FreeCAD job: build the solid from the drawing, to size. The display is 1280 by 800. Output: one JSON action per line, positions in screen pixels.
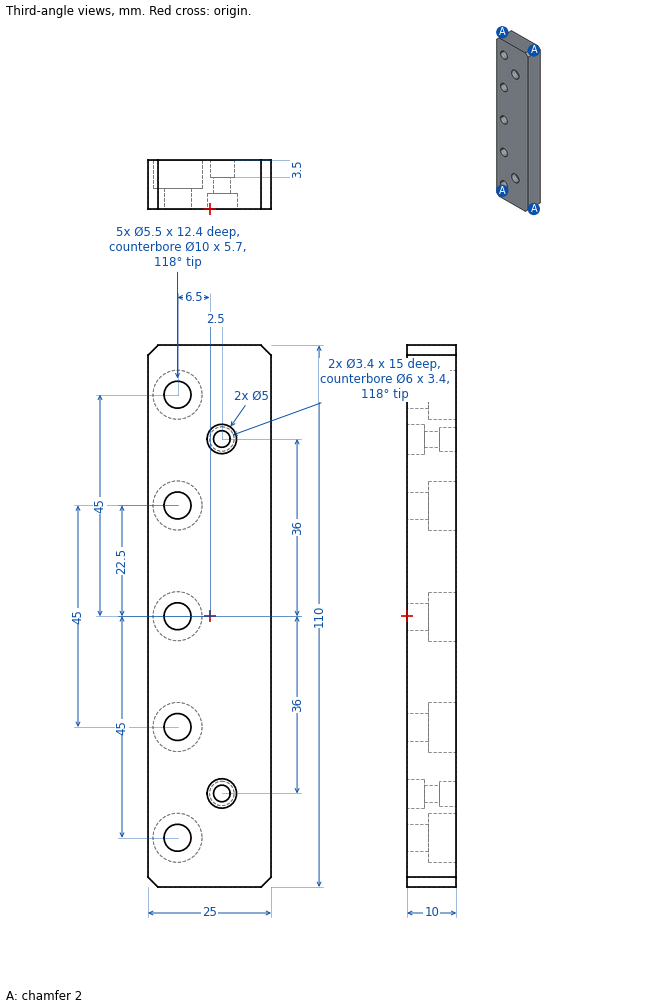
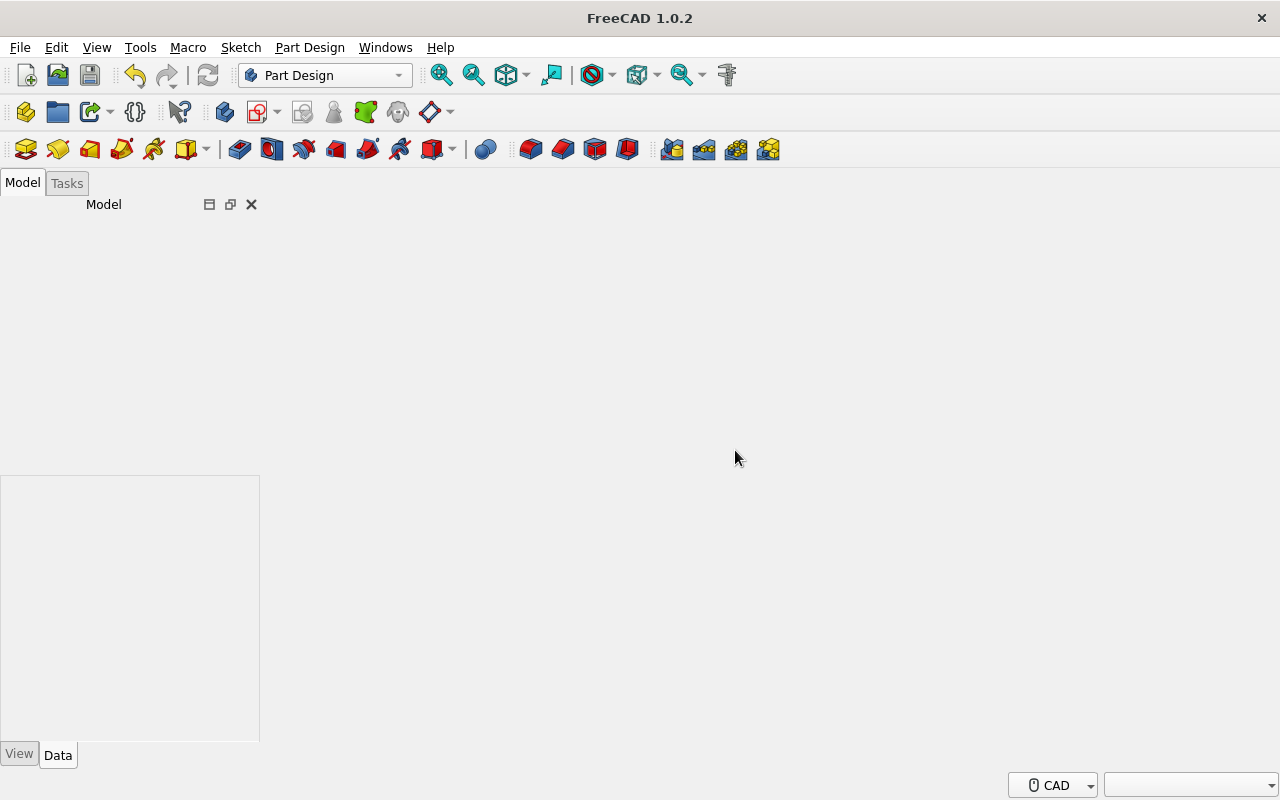
{"action": "left_click", "coordinate": [26, 76]}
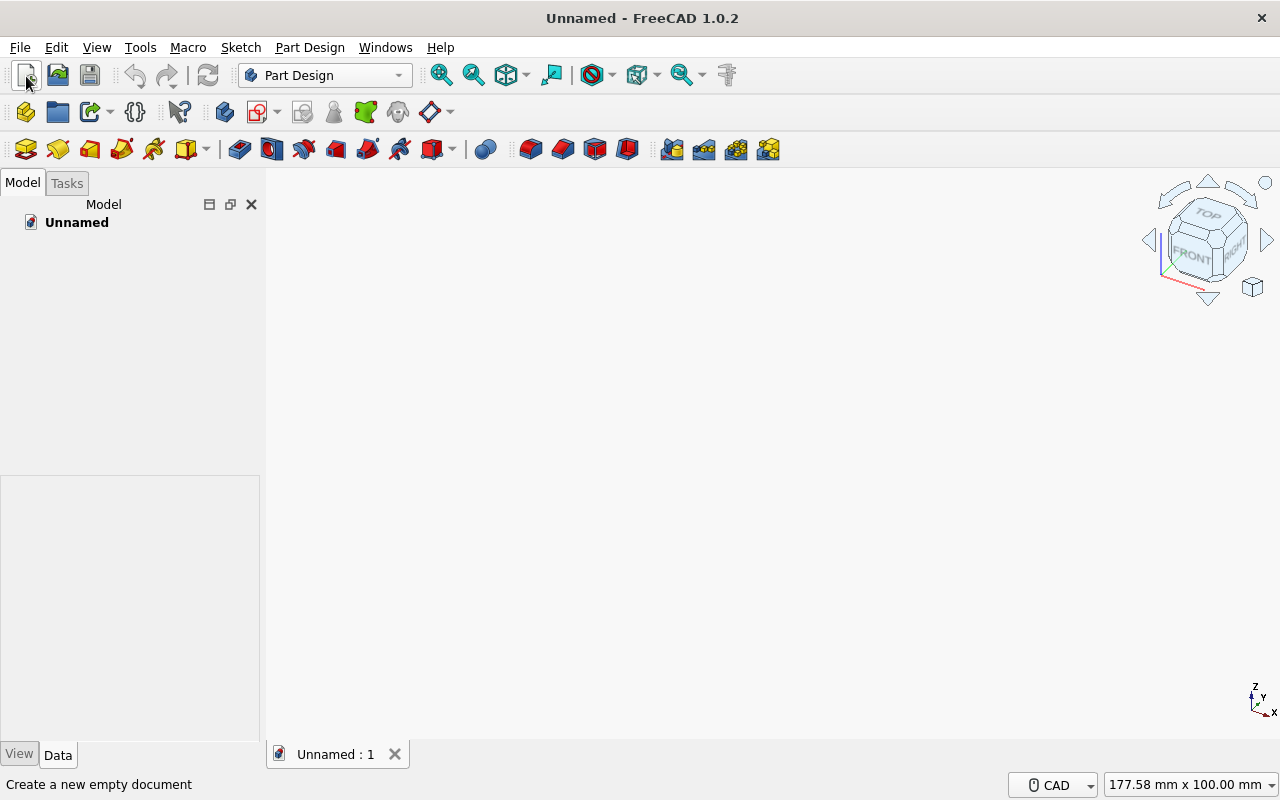
{"action": "left_click", "coordinate": [258, 112]}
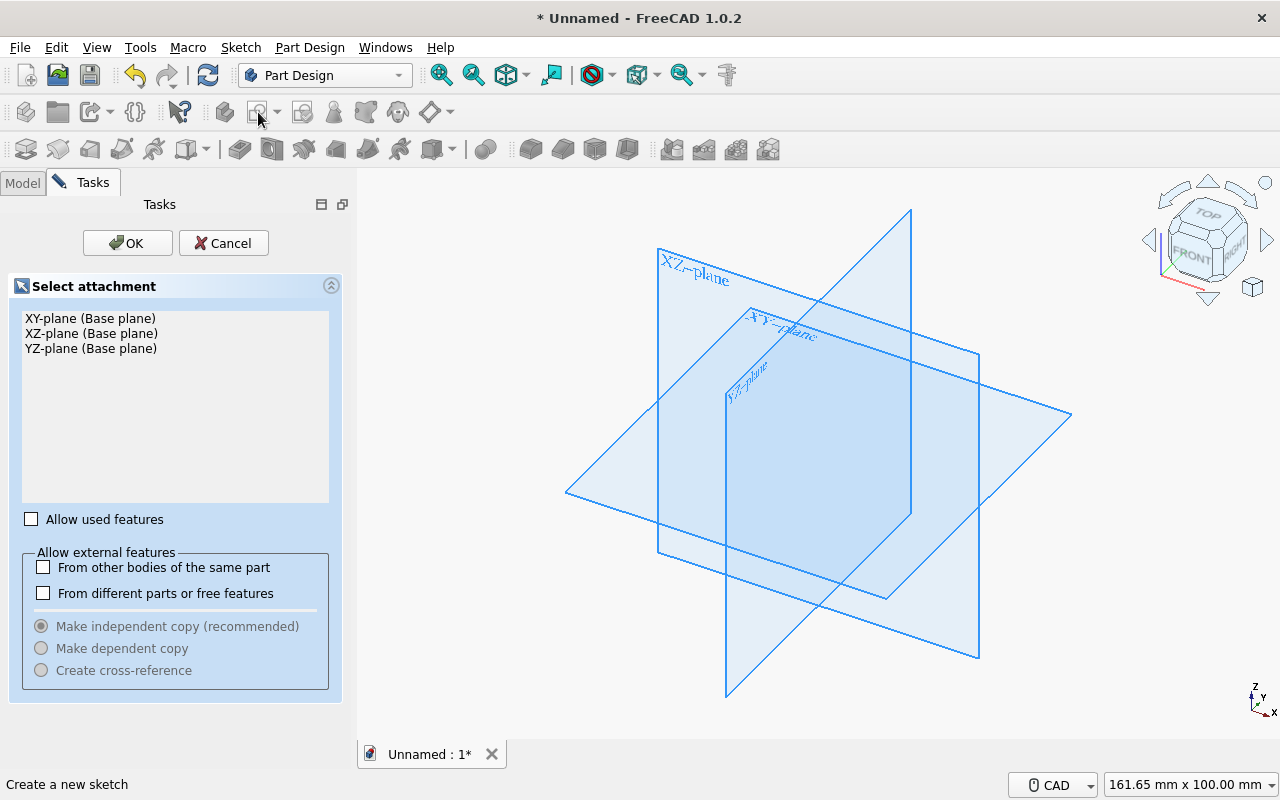
{"action": "left_click", "coordinate": [82, 334]}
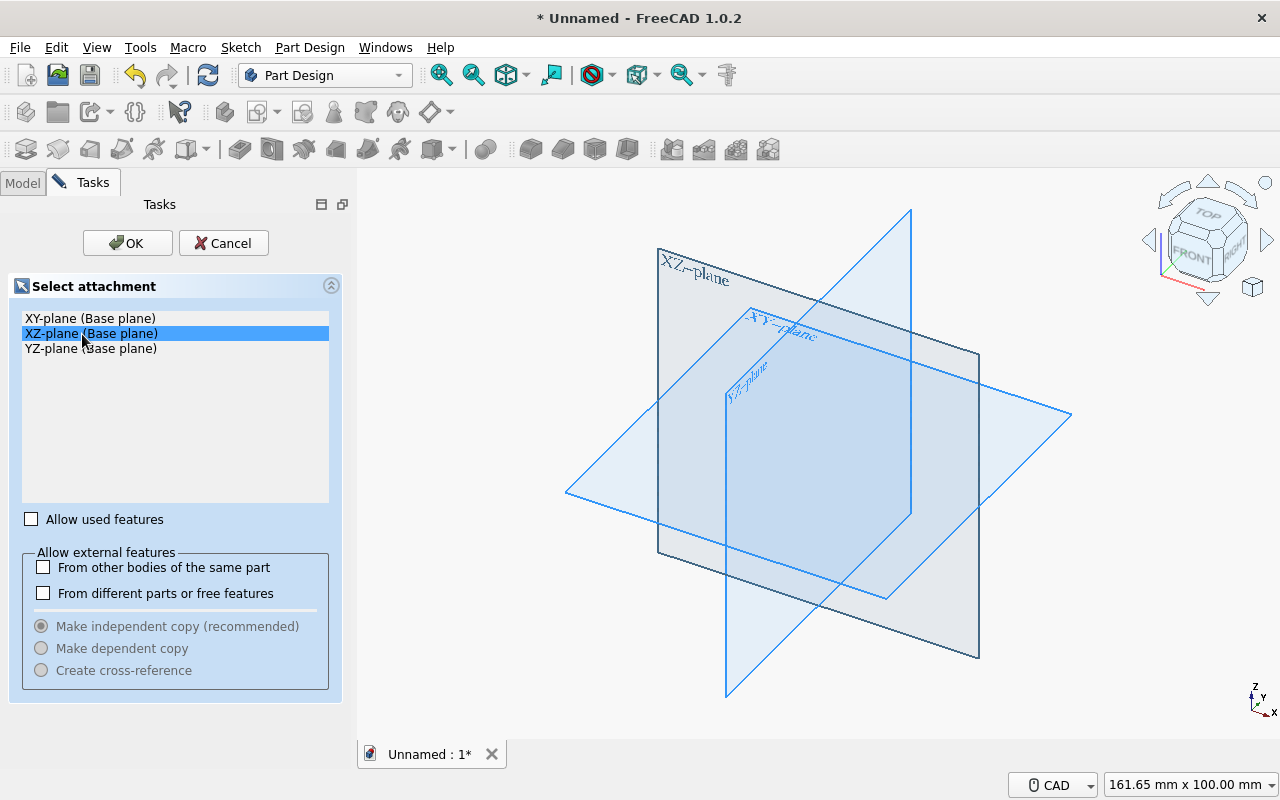
{"action": "left_click", "coordinate": [128, 243]}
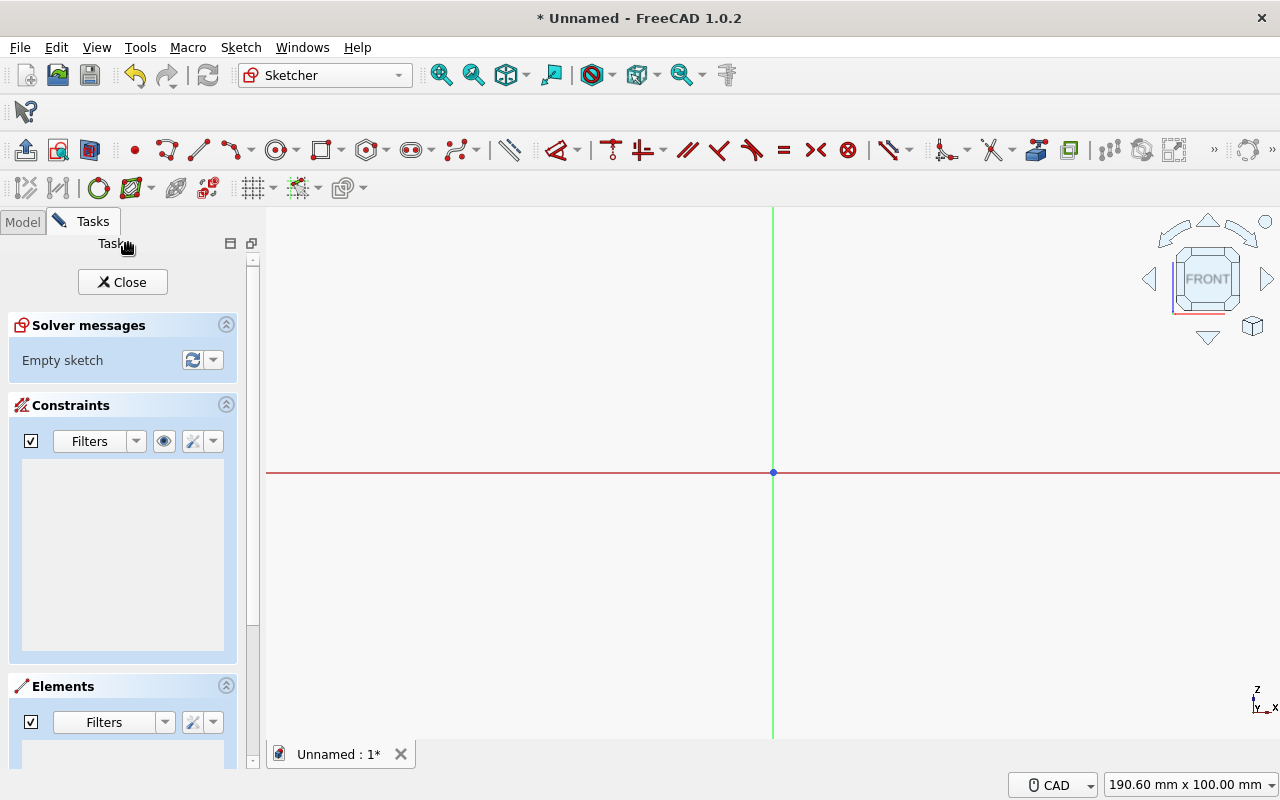
{"action": "scroll", "coordinate": [621, 473], "scroll_direction": "down", "scroll_amount": 3}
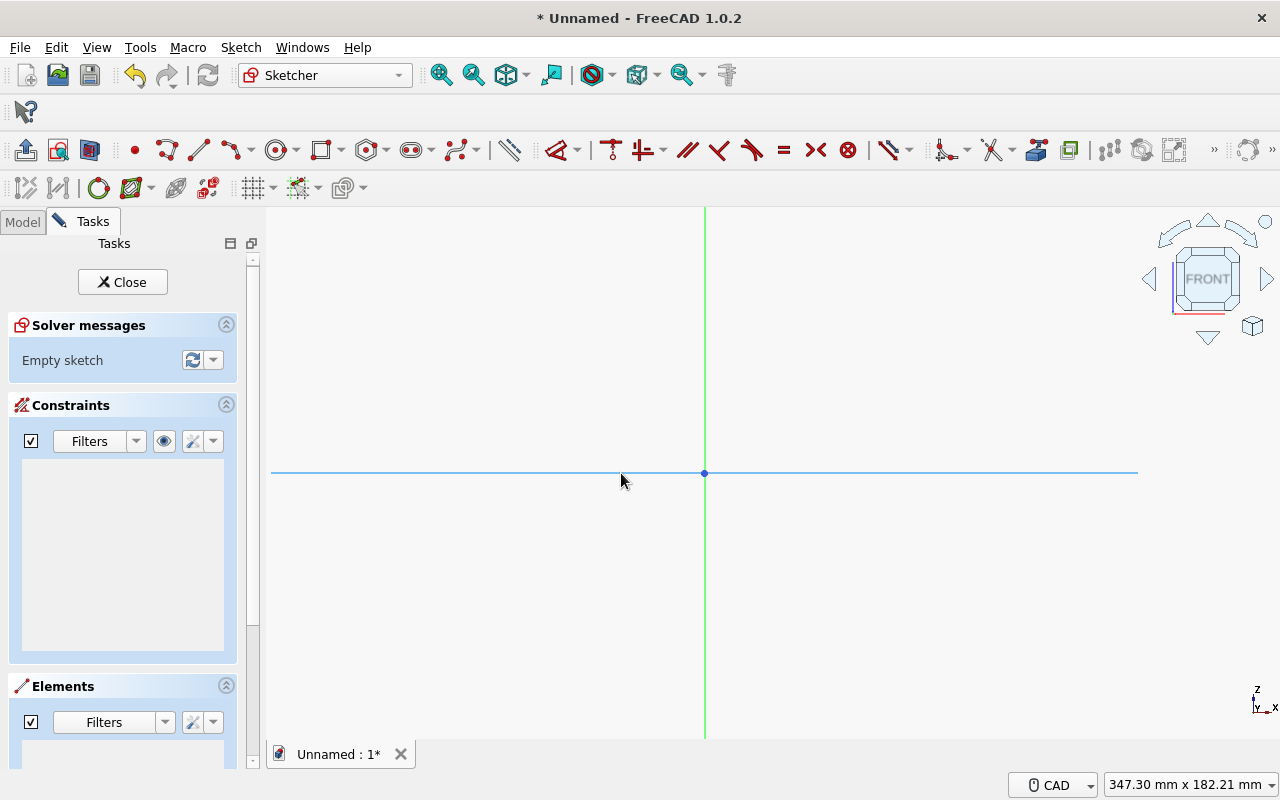
{"action": "left_click", "coordinate": [344, 150]}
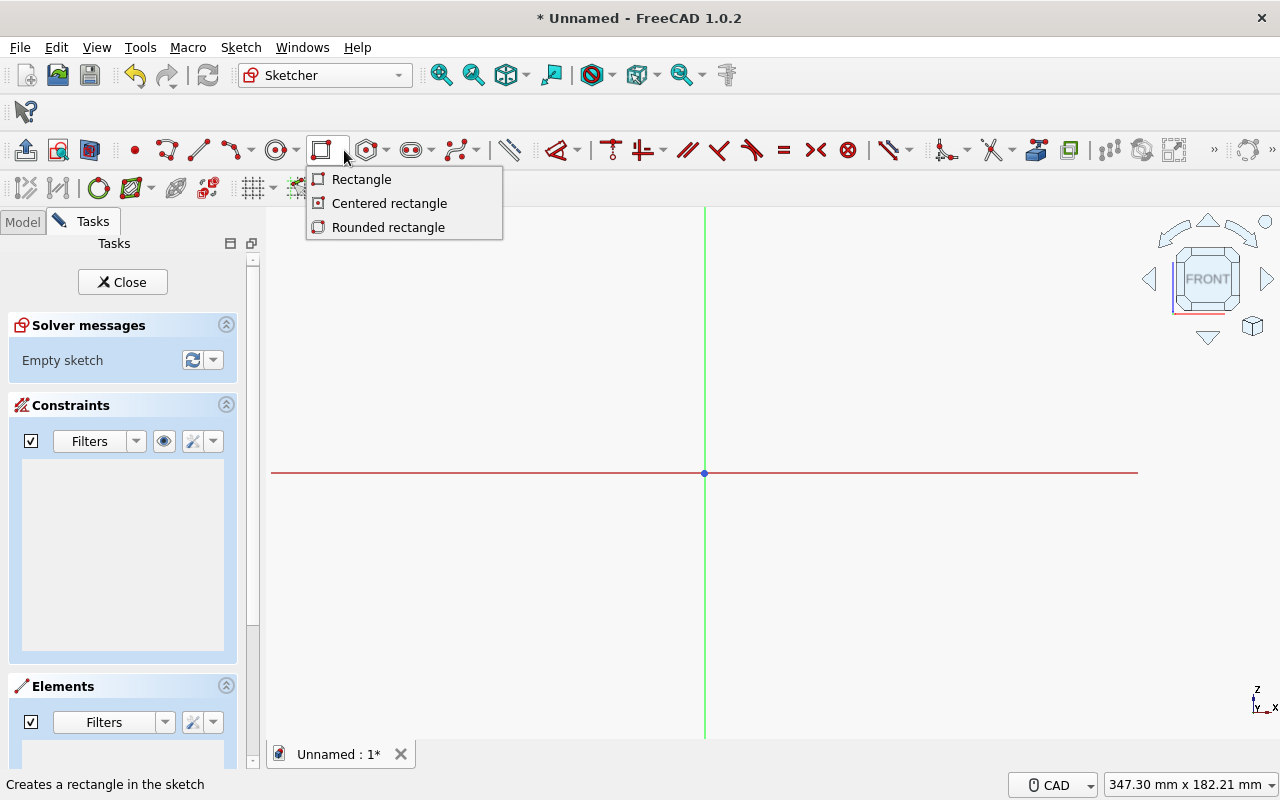
{"action": "left_click", "coordinate": [404, 203]}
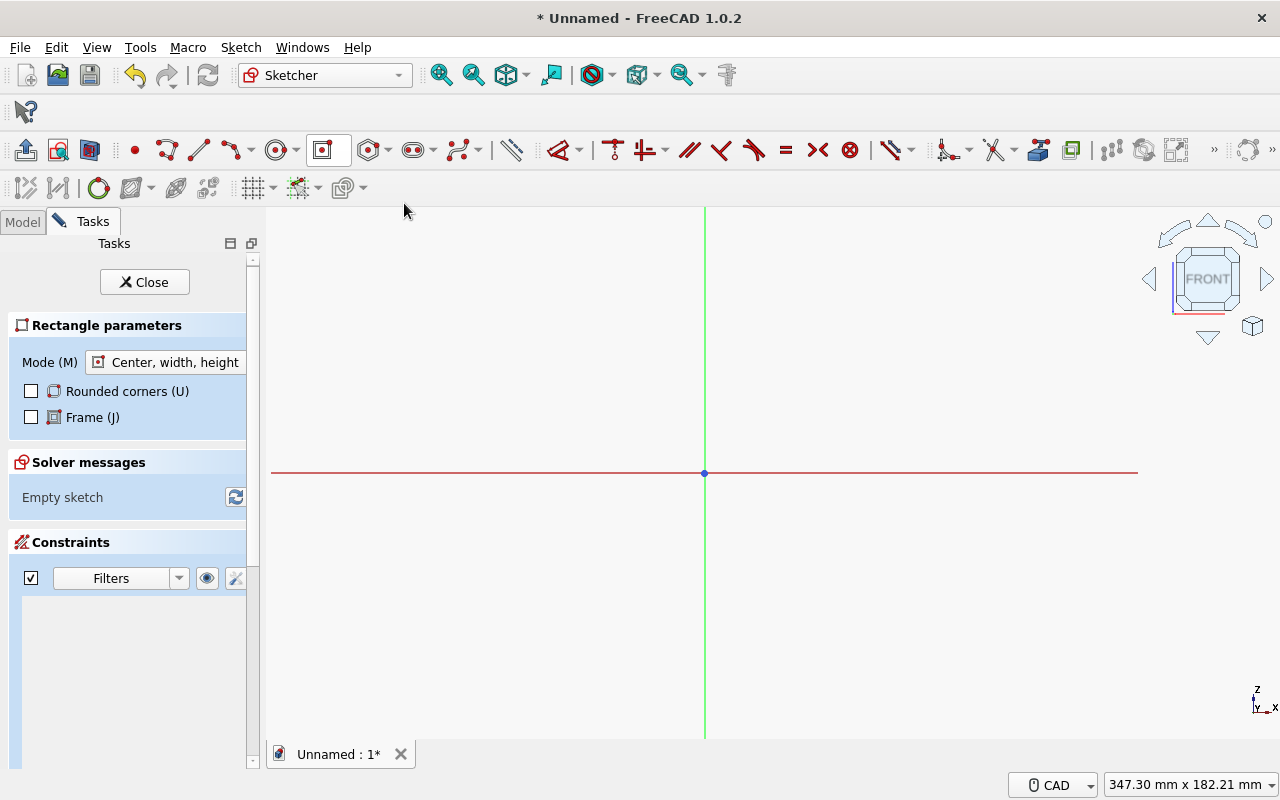
{"action": "left_click", "coordinate": [705, 473]}
{"action": "mouse_move", "coordinate": [741, 313]}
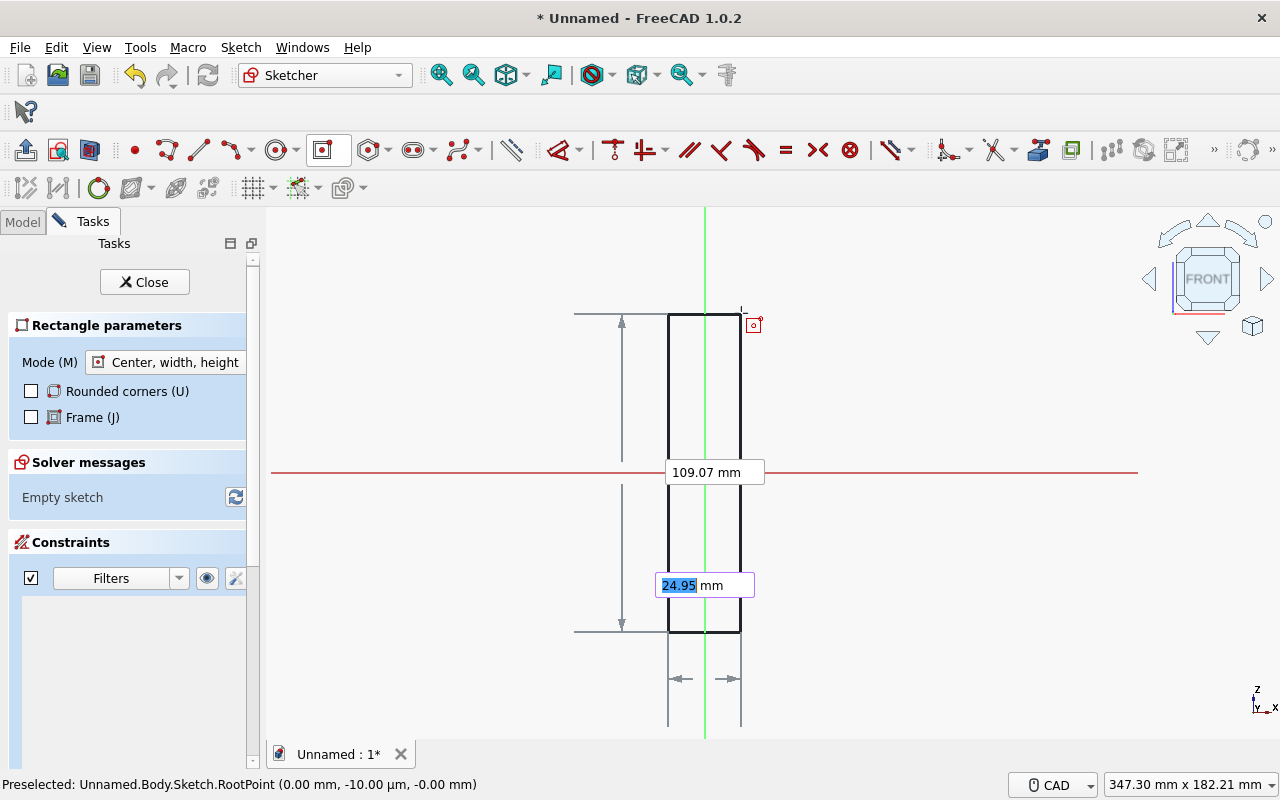
{"action": "type", "text": "25"}
{"action": "key", "text": "Tab"}
{"action": "type", "text": "110"}
{"action": "key", "text": "Return"}
{"action": "key", "text": "Escape"}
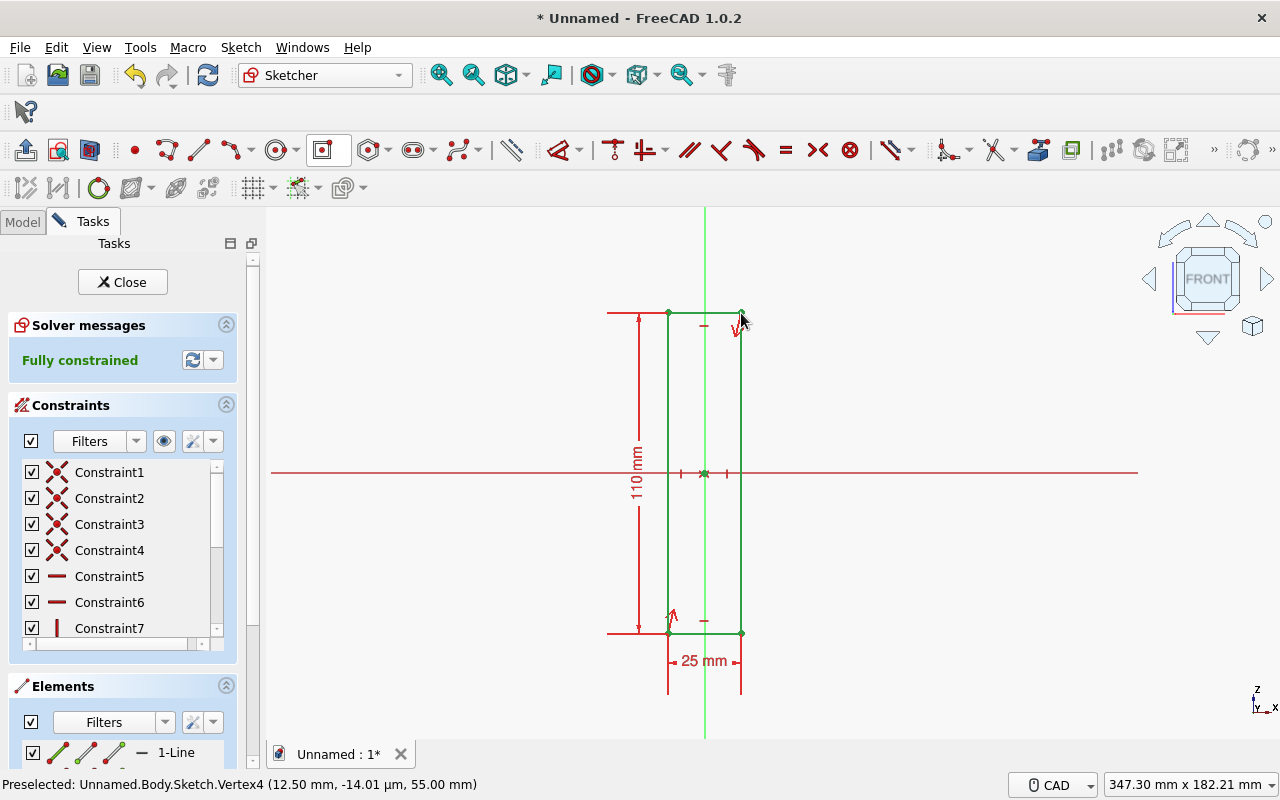
{"action": "left_click", "coordinate": [123, 282]}